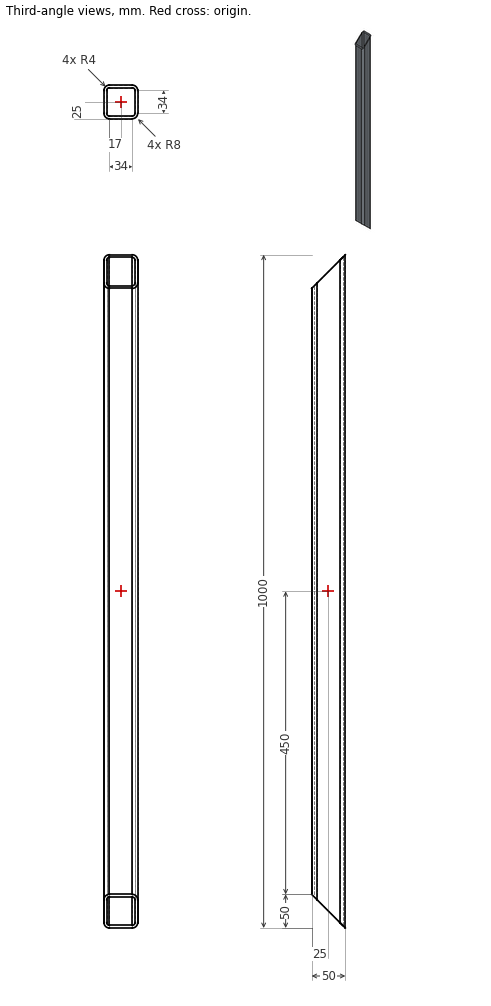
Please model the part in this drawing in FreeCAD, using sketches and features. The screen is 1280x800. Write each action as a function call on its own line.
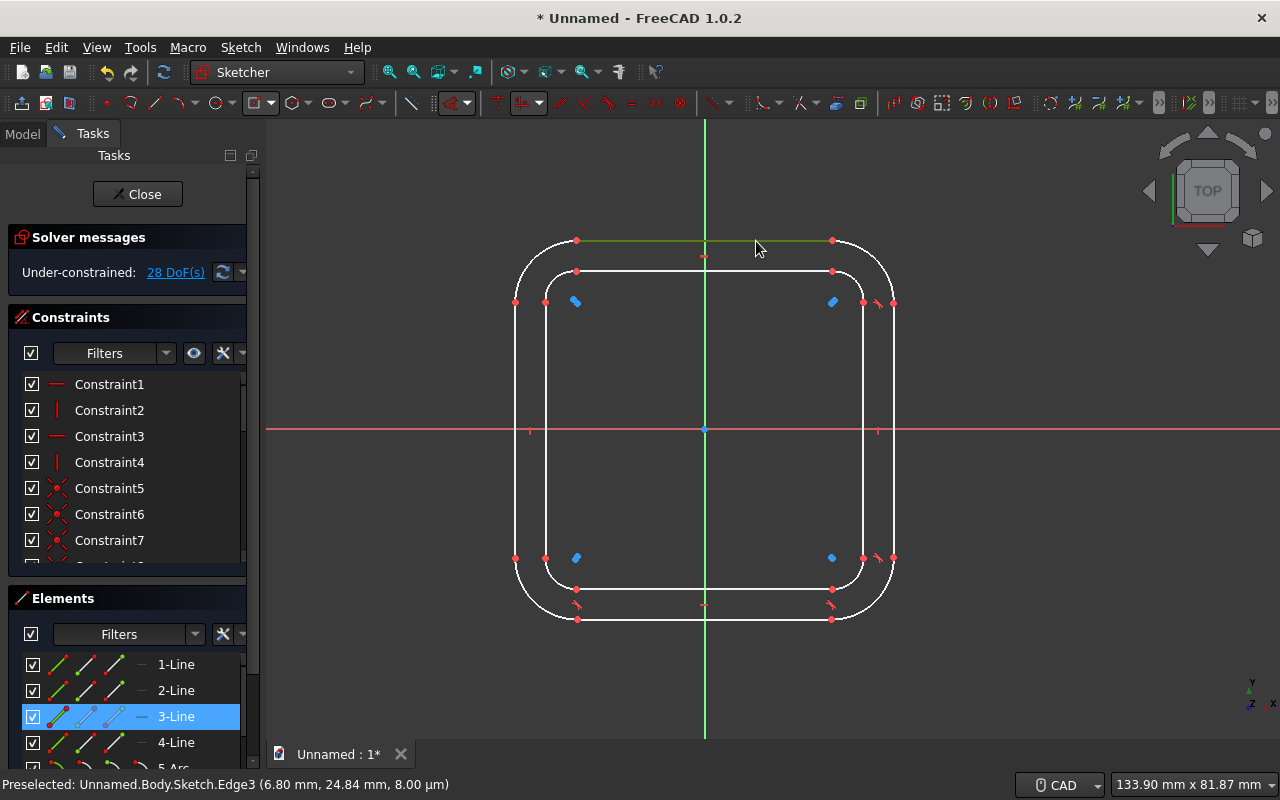
click(887, 276)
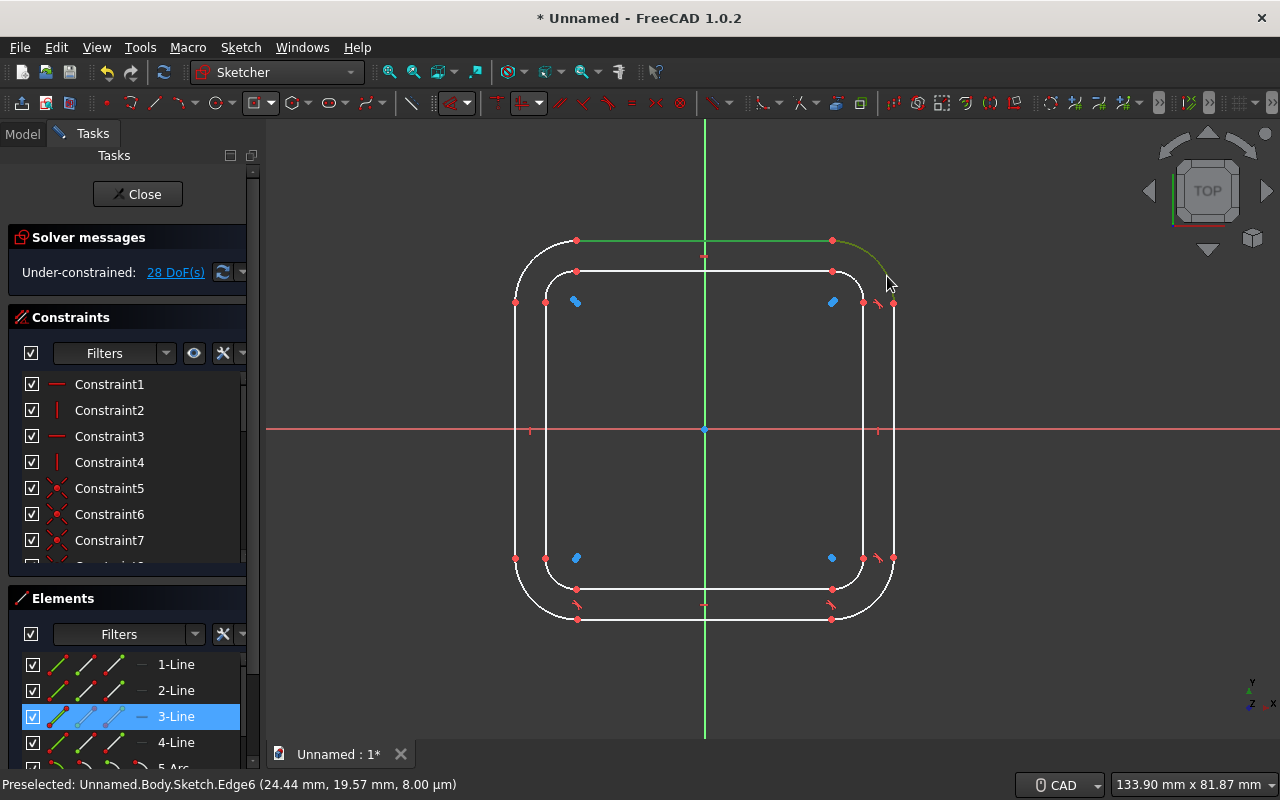
key(t)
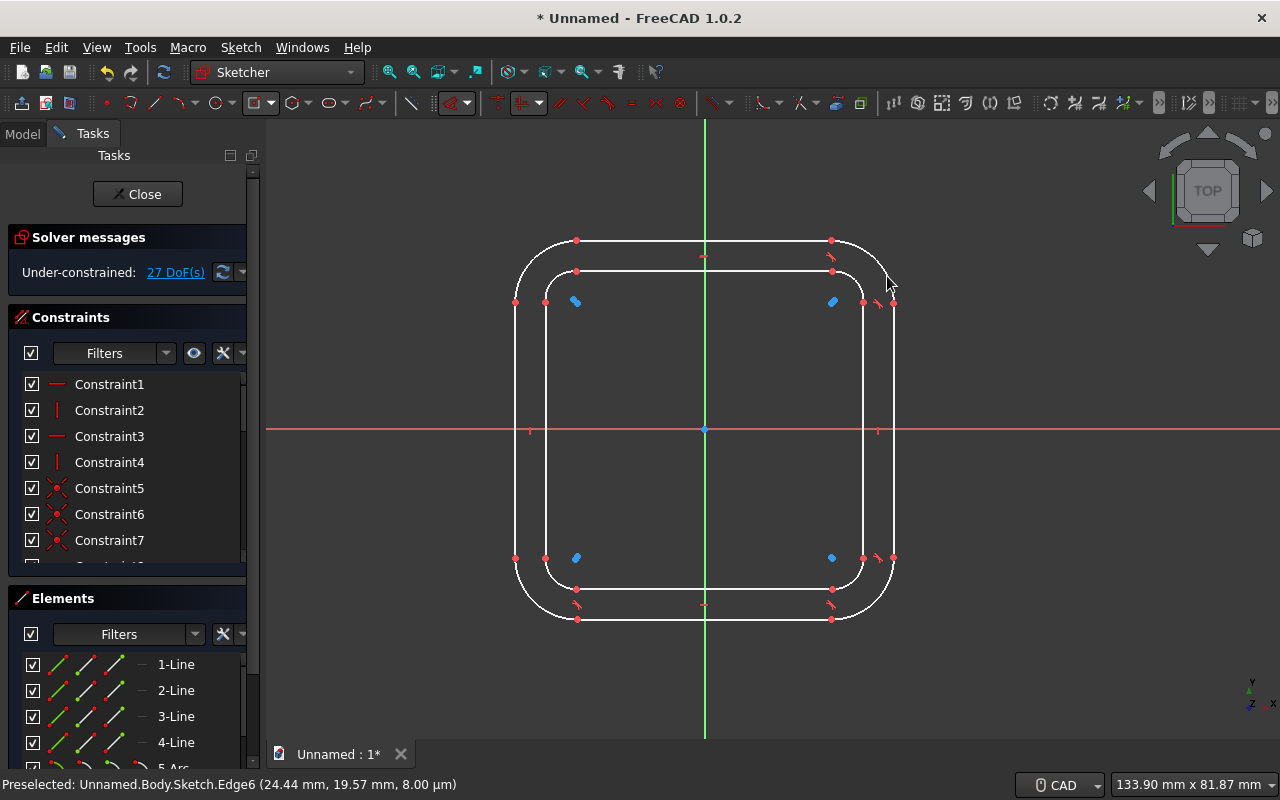
click(755, 241)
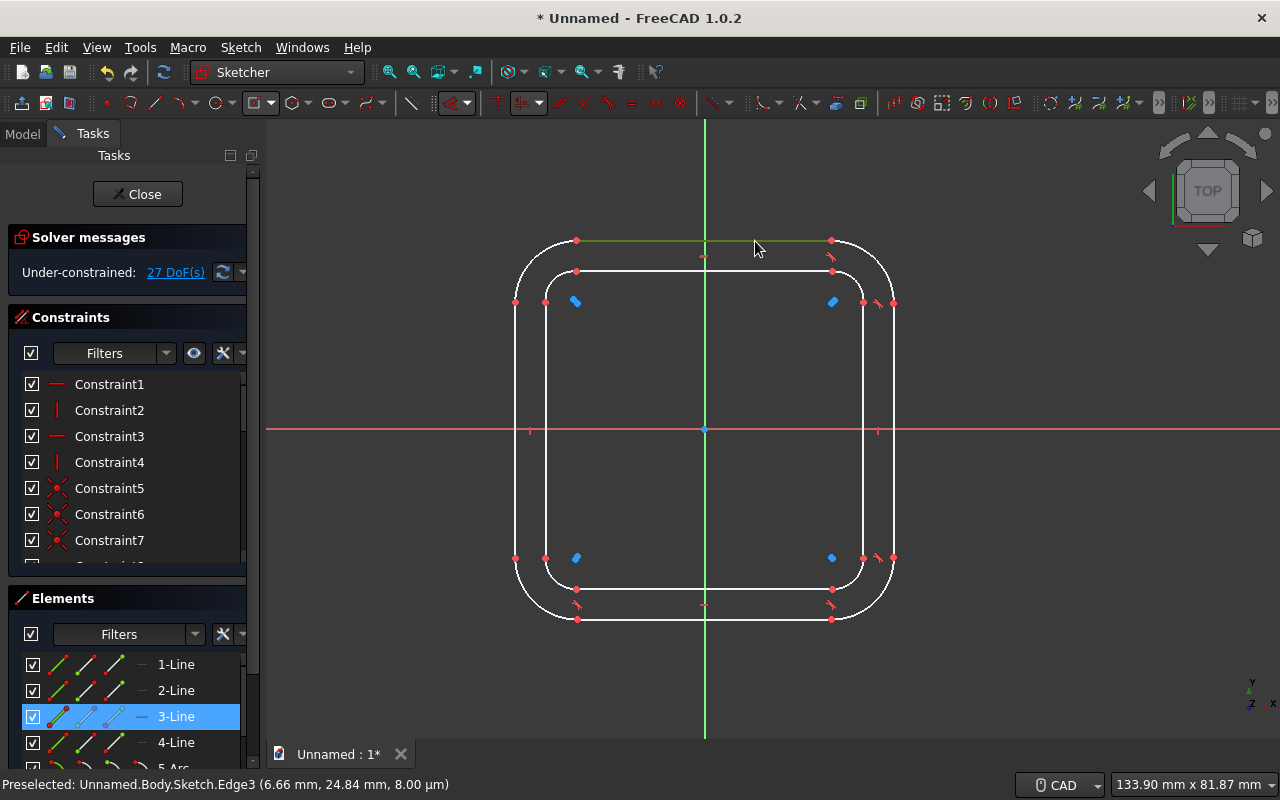
click(549, 248)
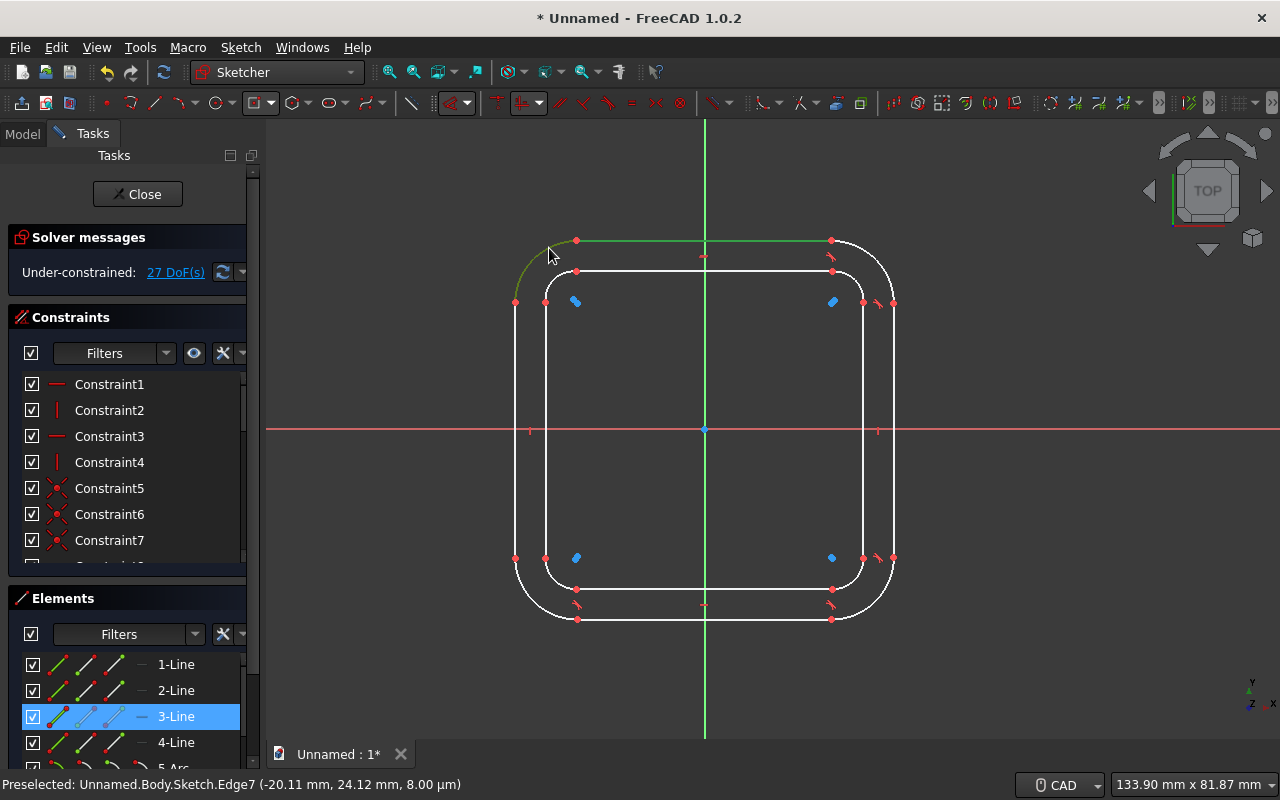
click(608, 104)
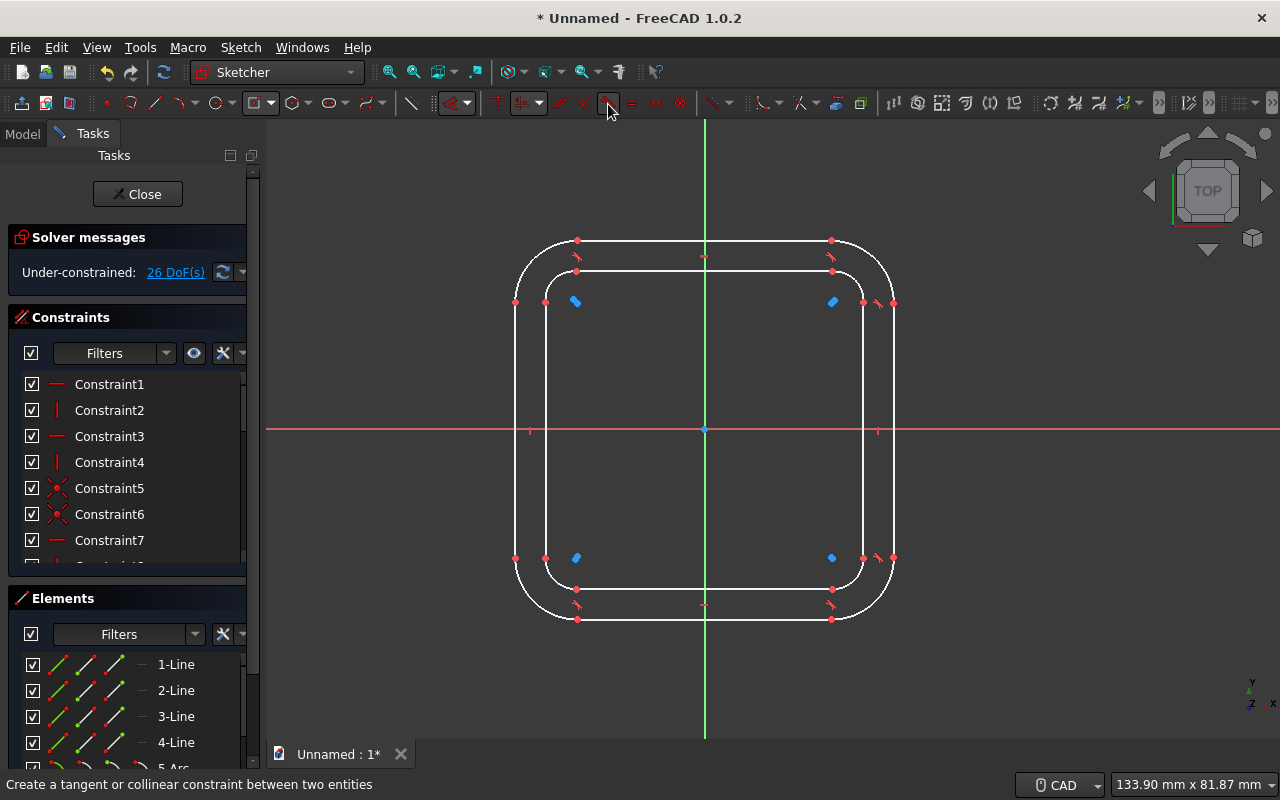
click(515, 379)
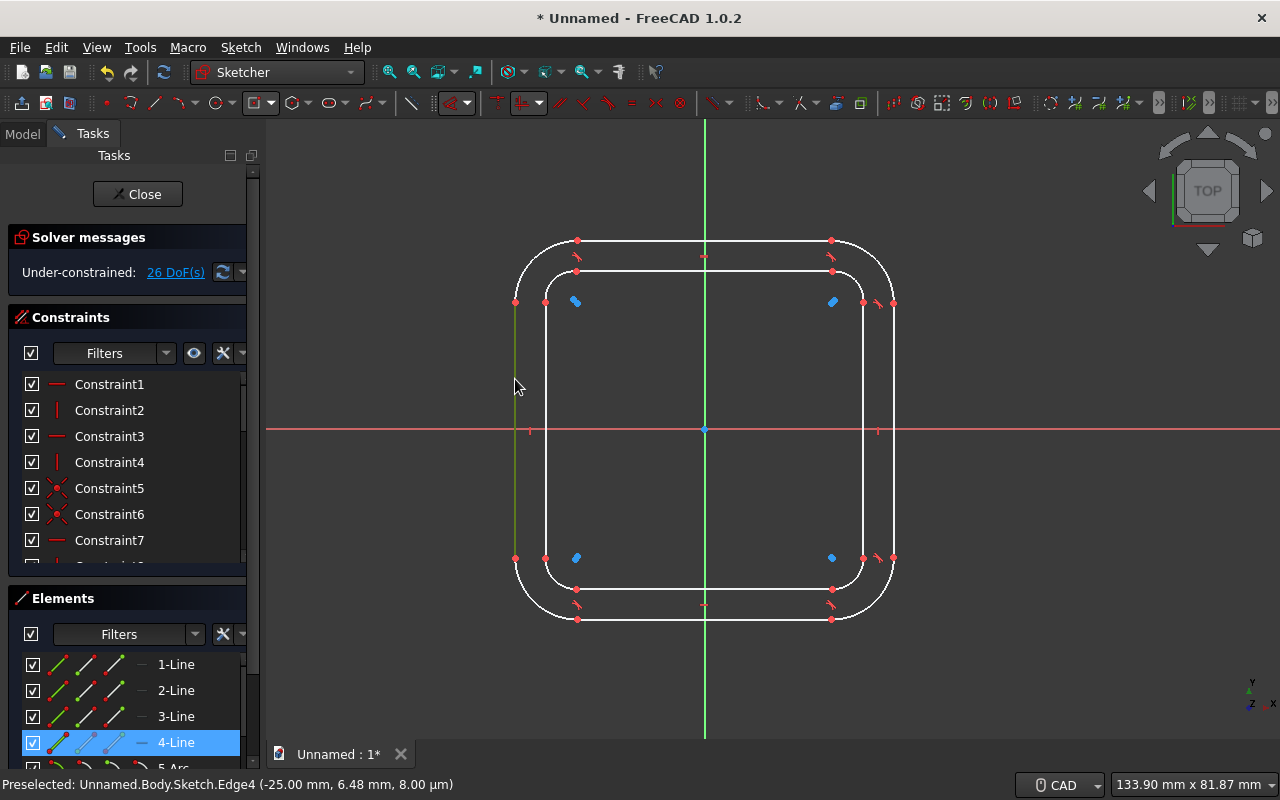
click(550, 248)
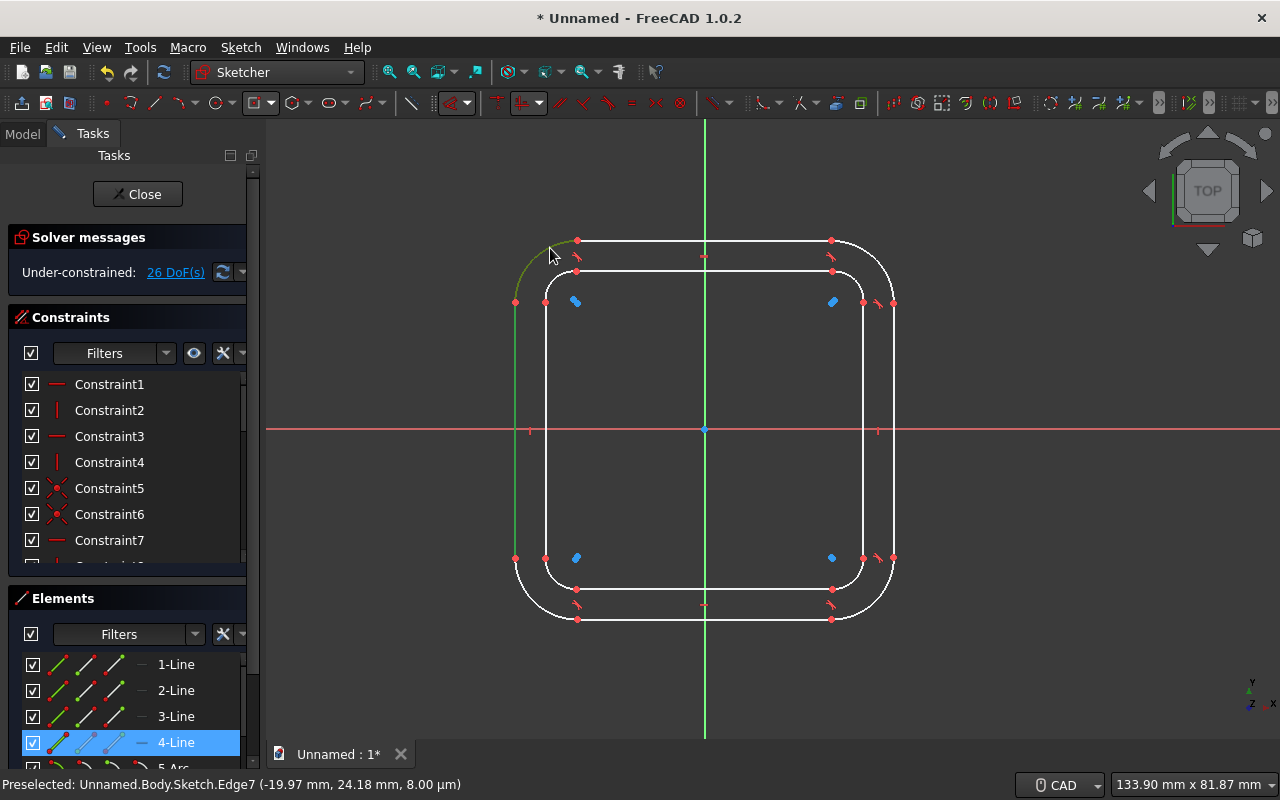
key(t)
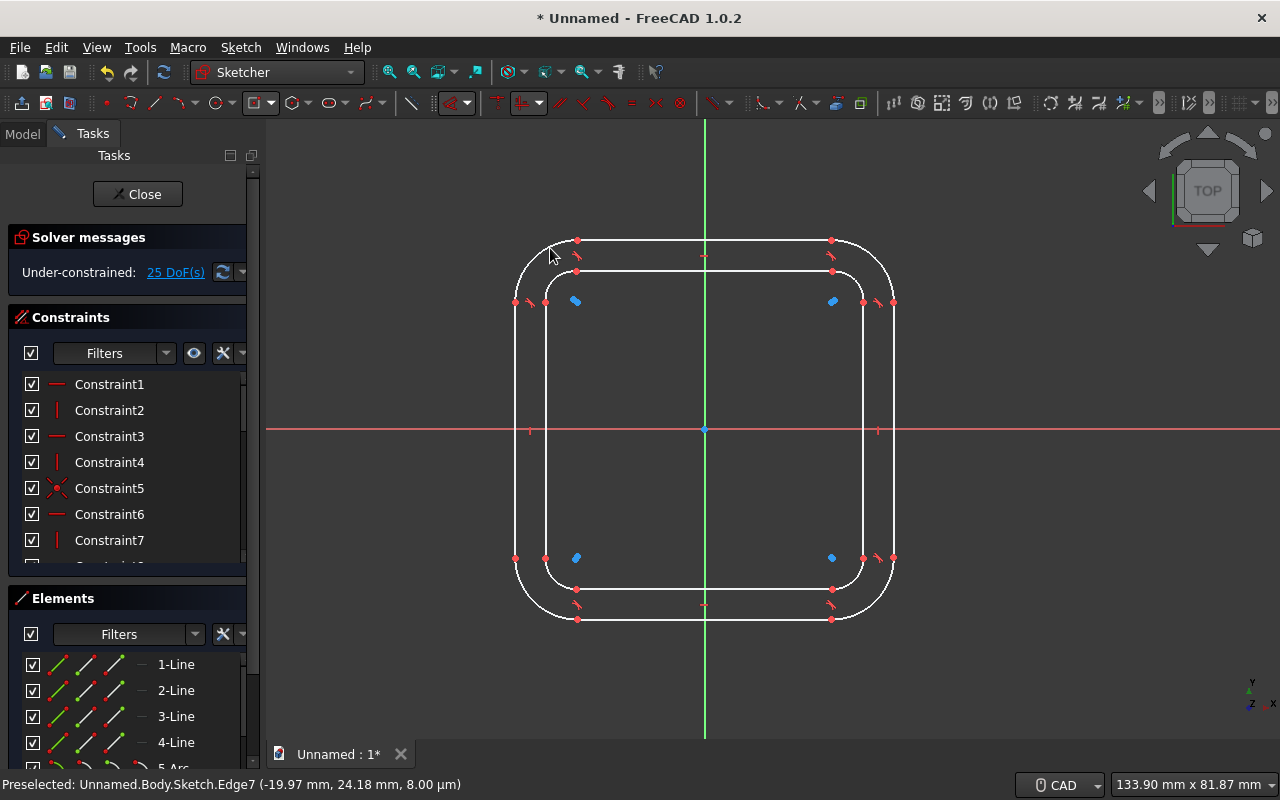
click(515, 379)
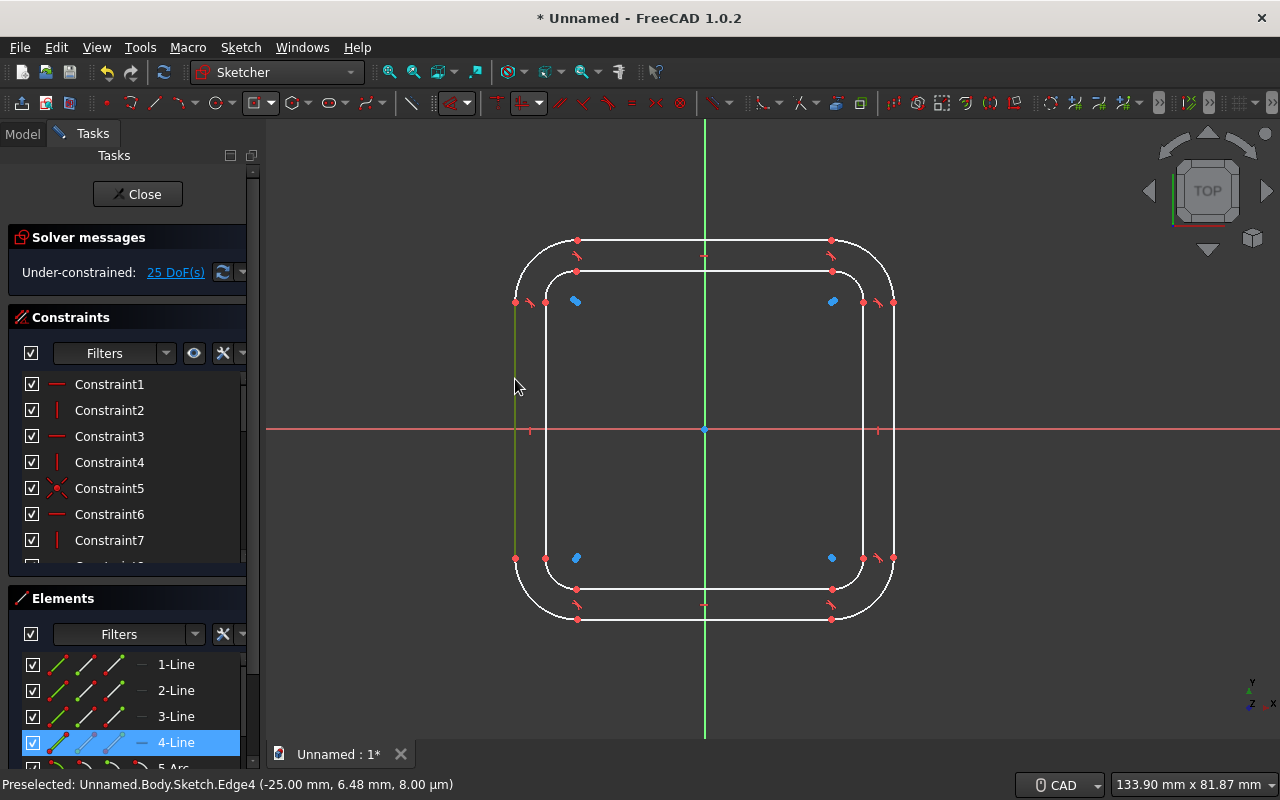
click(523, 586)